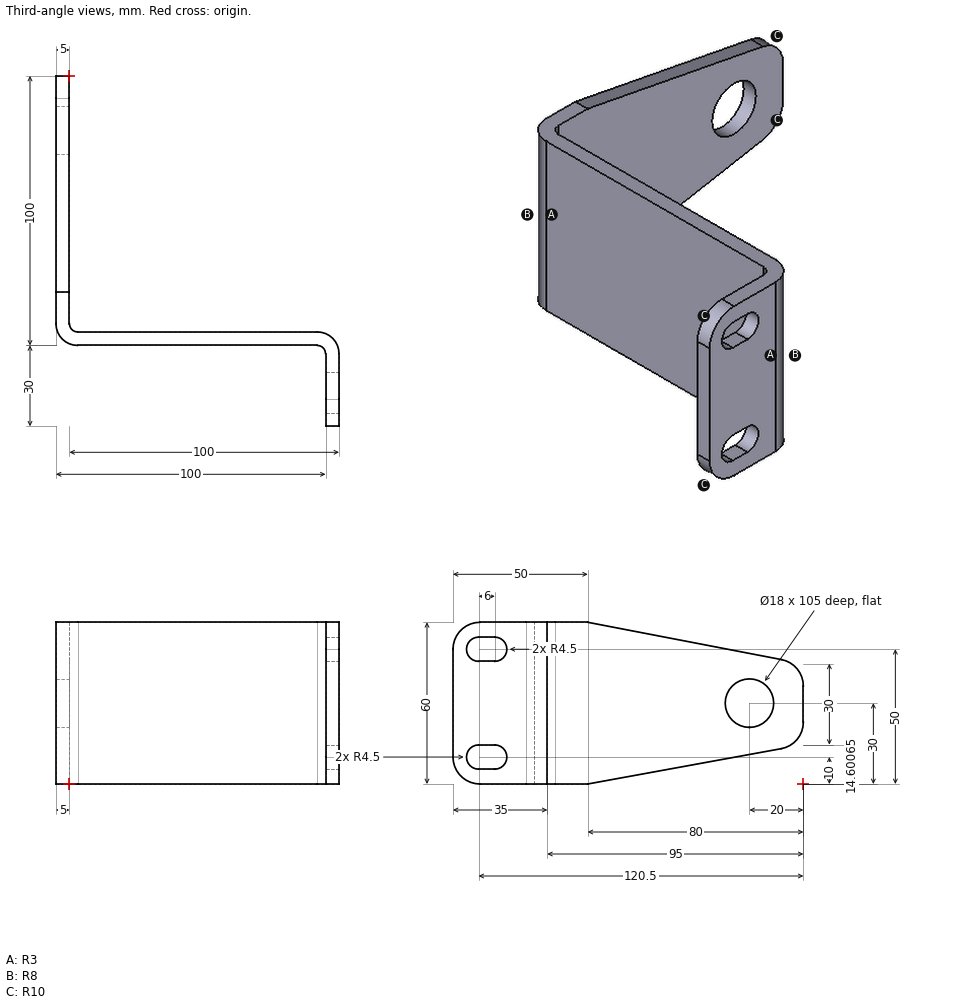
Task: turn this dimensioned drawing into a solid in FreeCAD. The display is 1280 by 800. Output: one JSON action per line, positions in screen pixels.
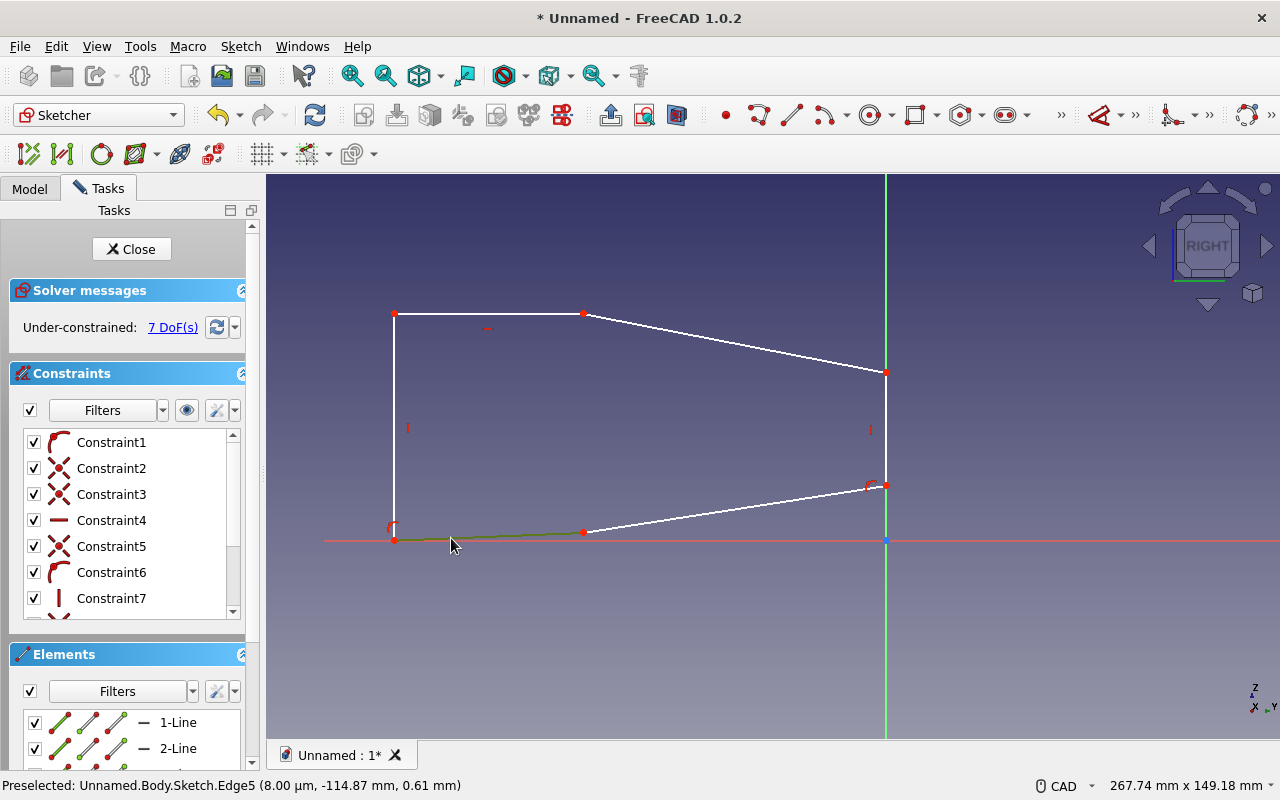
{"action": "key", "text": "h"}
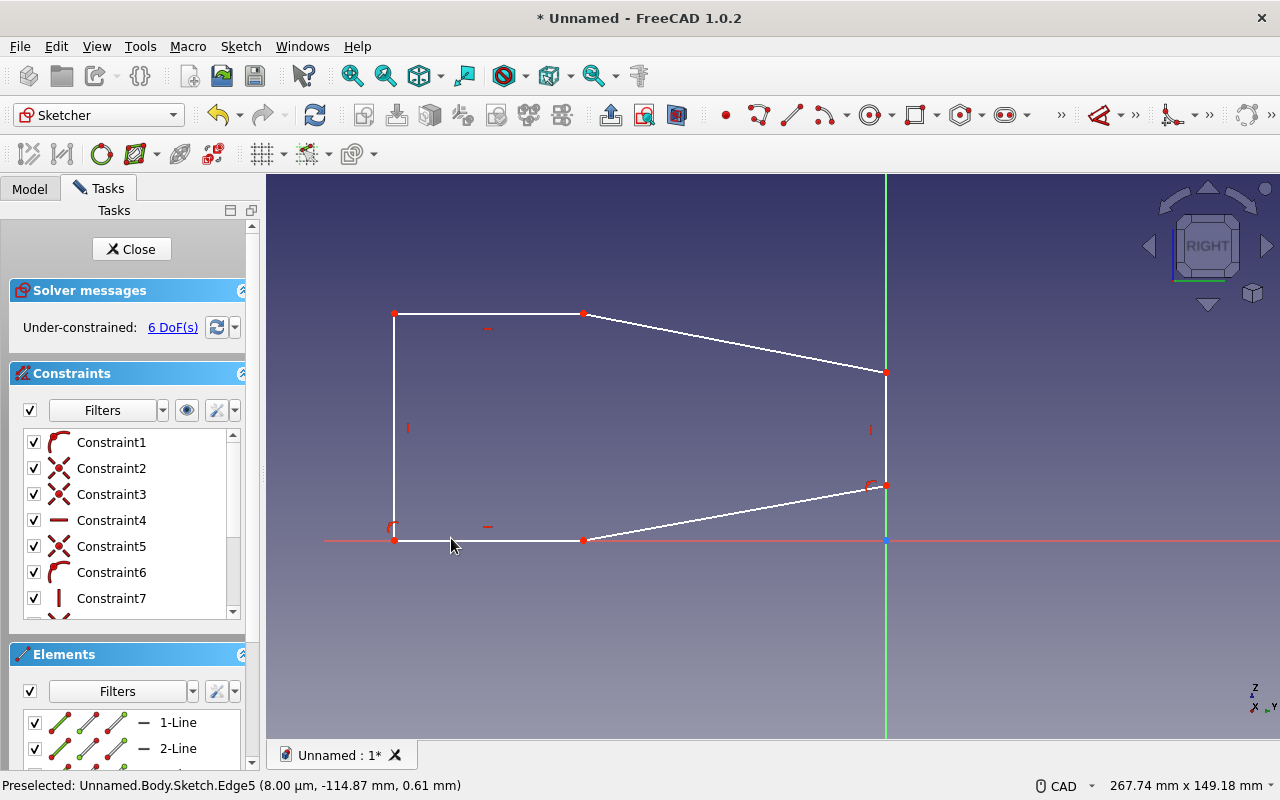
{"action": "left_click", "coordinate": [886, 452]}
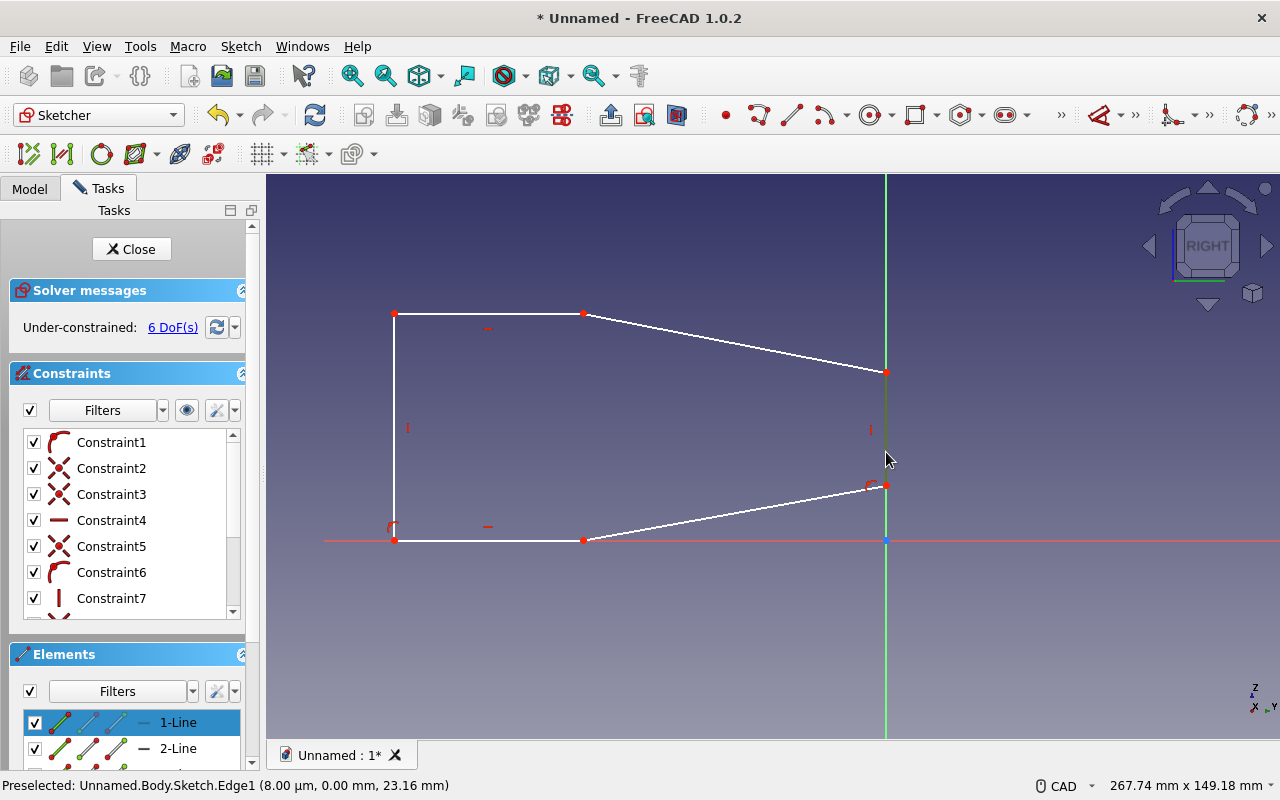
{"action": "left_click", "coordinate": [1120, 116]}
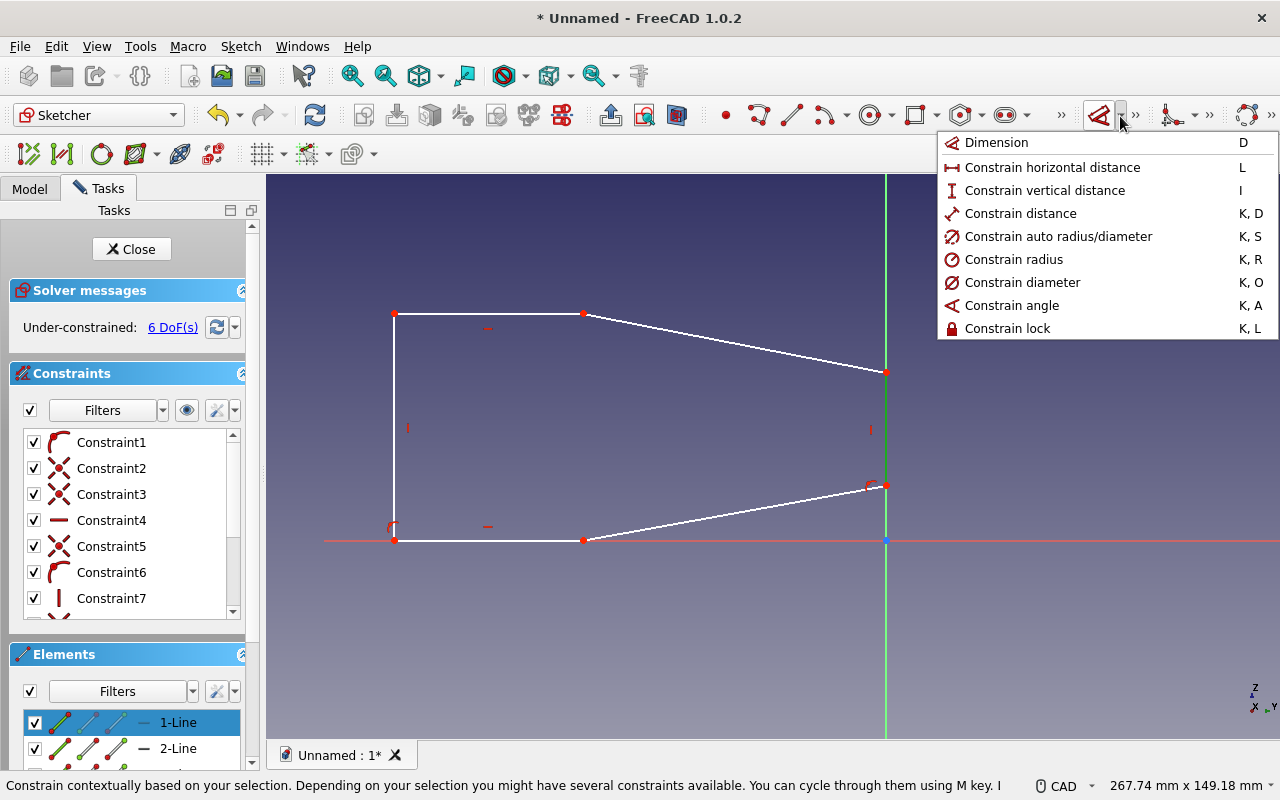
{"action": "left_click", "coordinate": [1108, 190]}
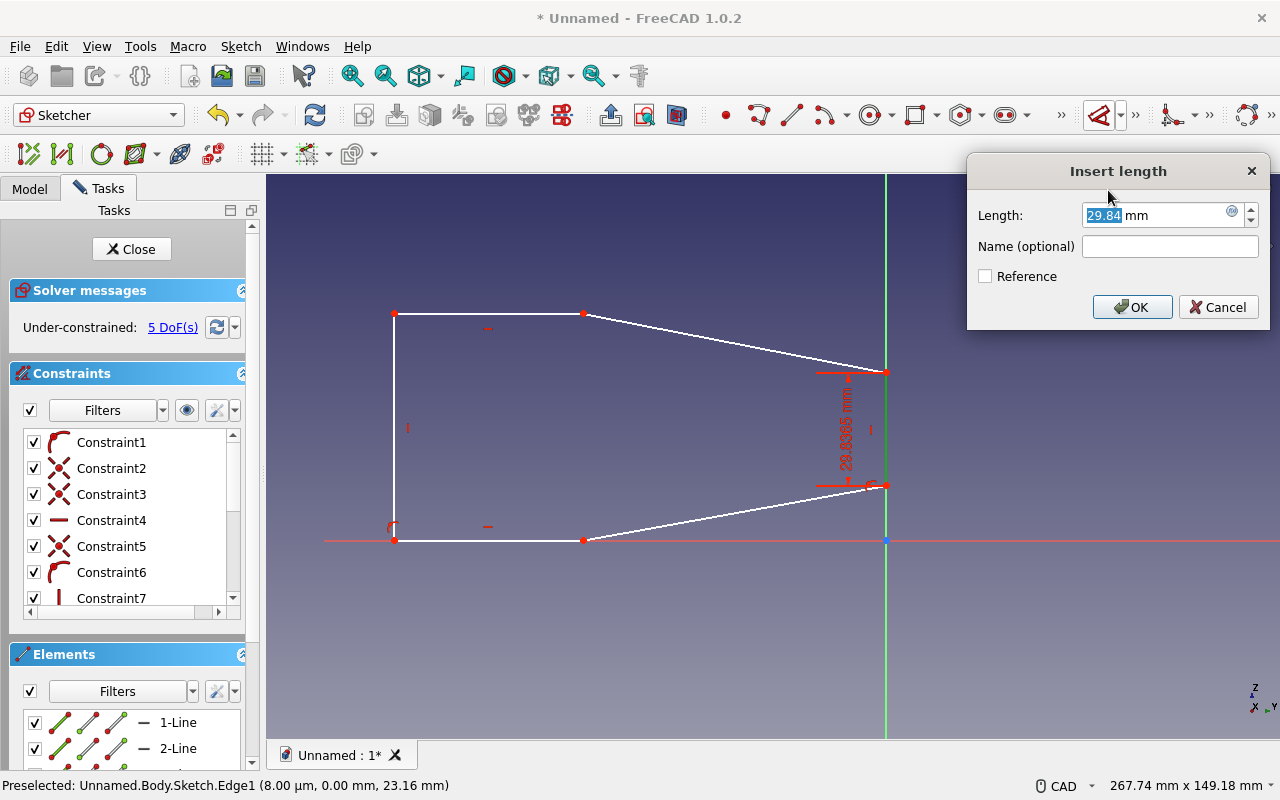
{"action": "type", "text": "30"}
{"action": "key", "text": "Return"}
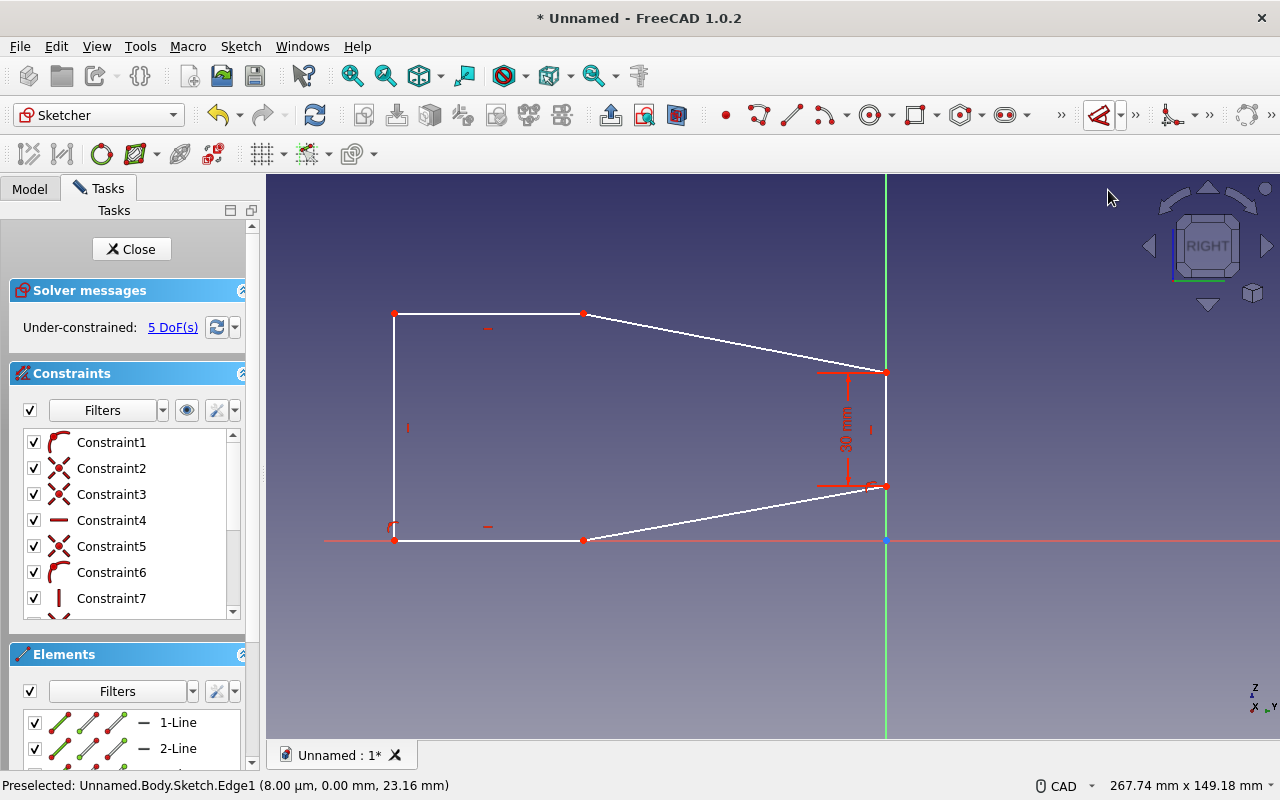
{"action": "left_click", "coordinate": [526, 314]}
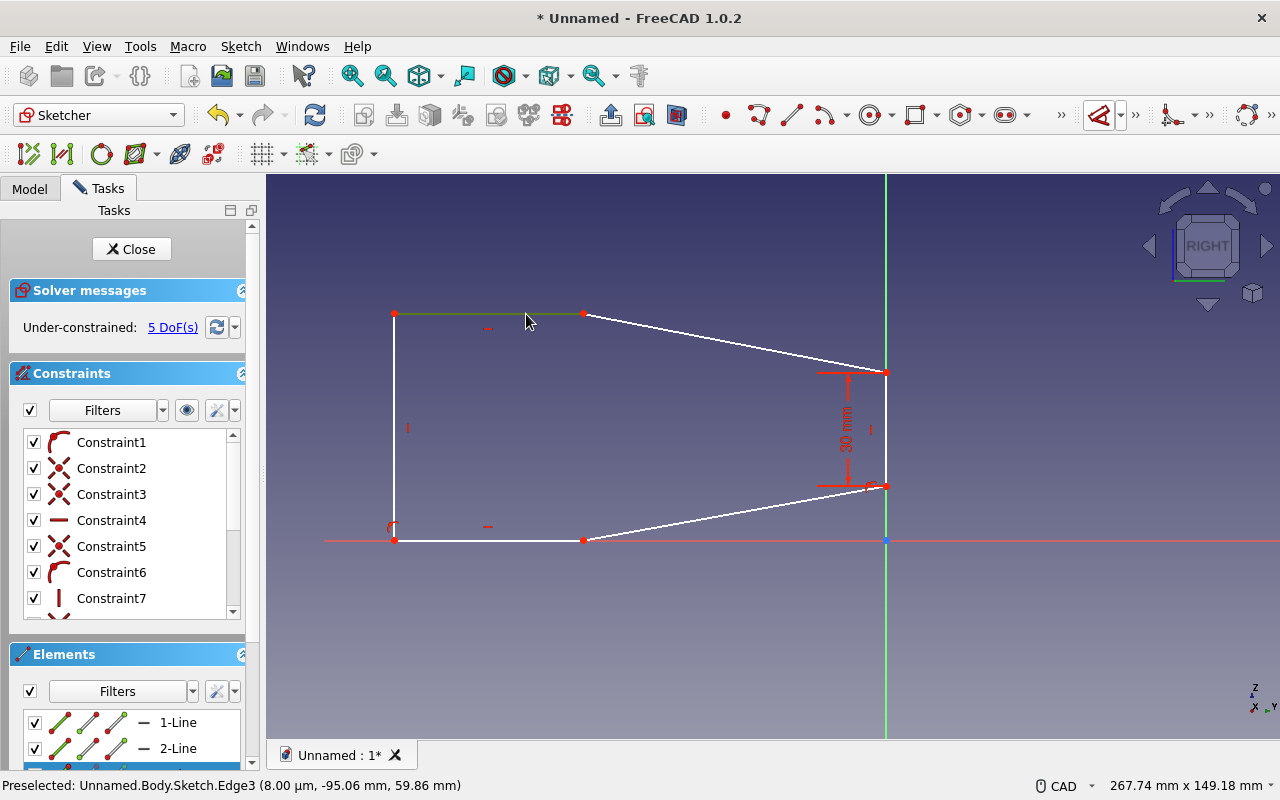
{"action": "key", "text": "l"}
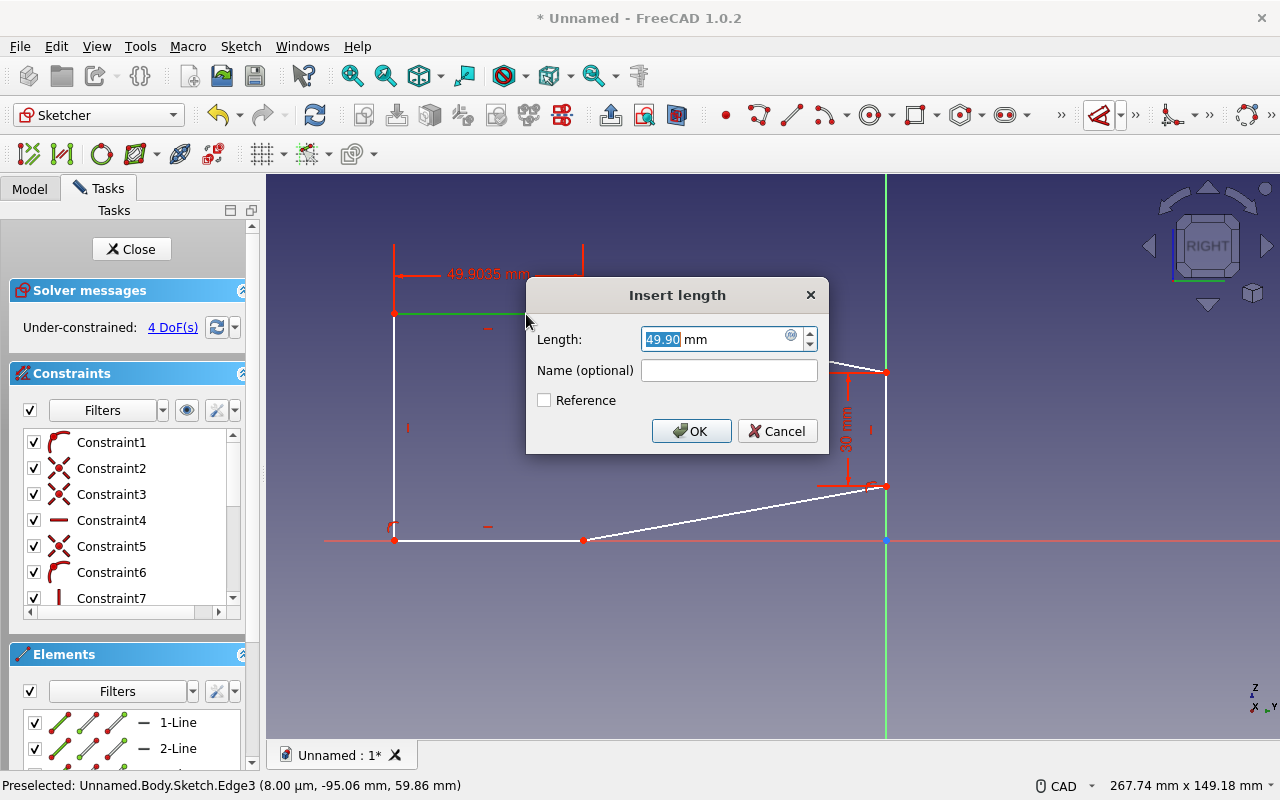
{"action": "type", "text": "50"}
{"action": "key", "text": "Return"}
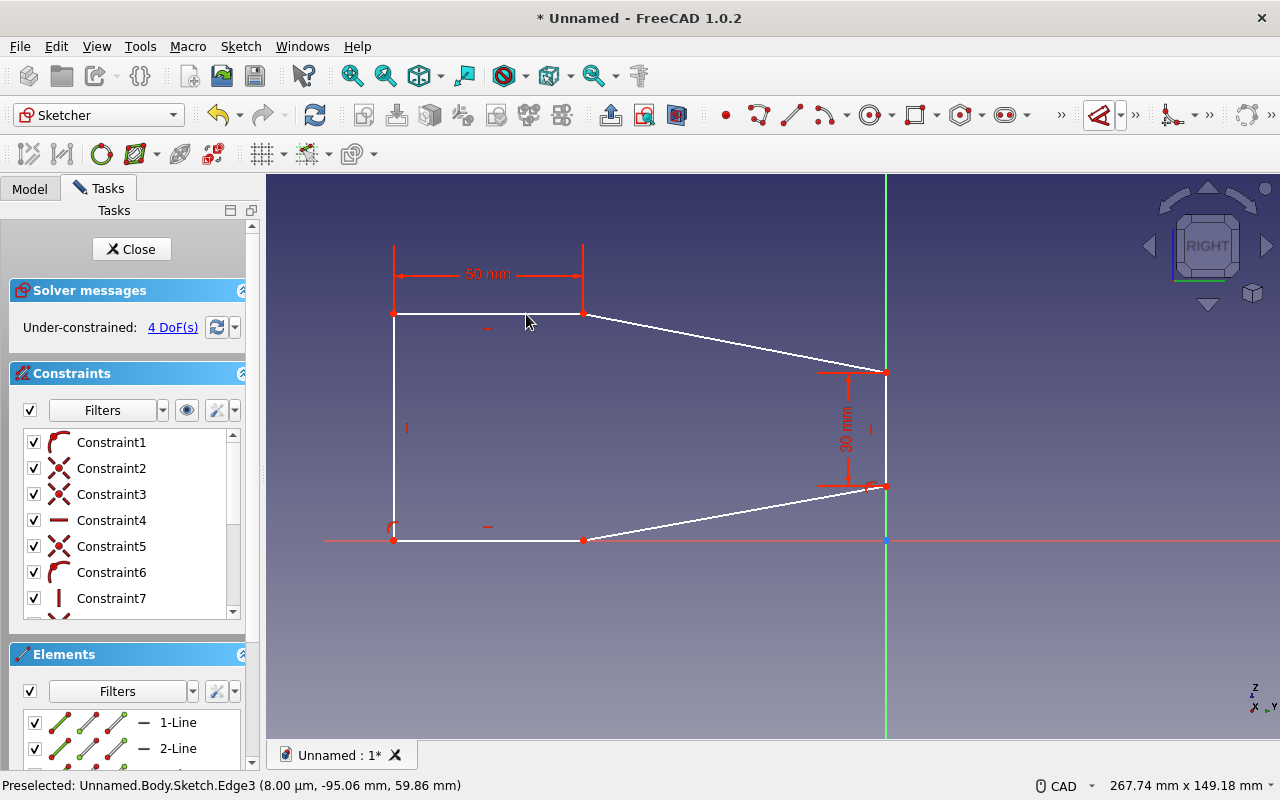
{"action": "left_click", "coordinate": [394, 382]}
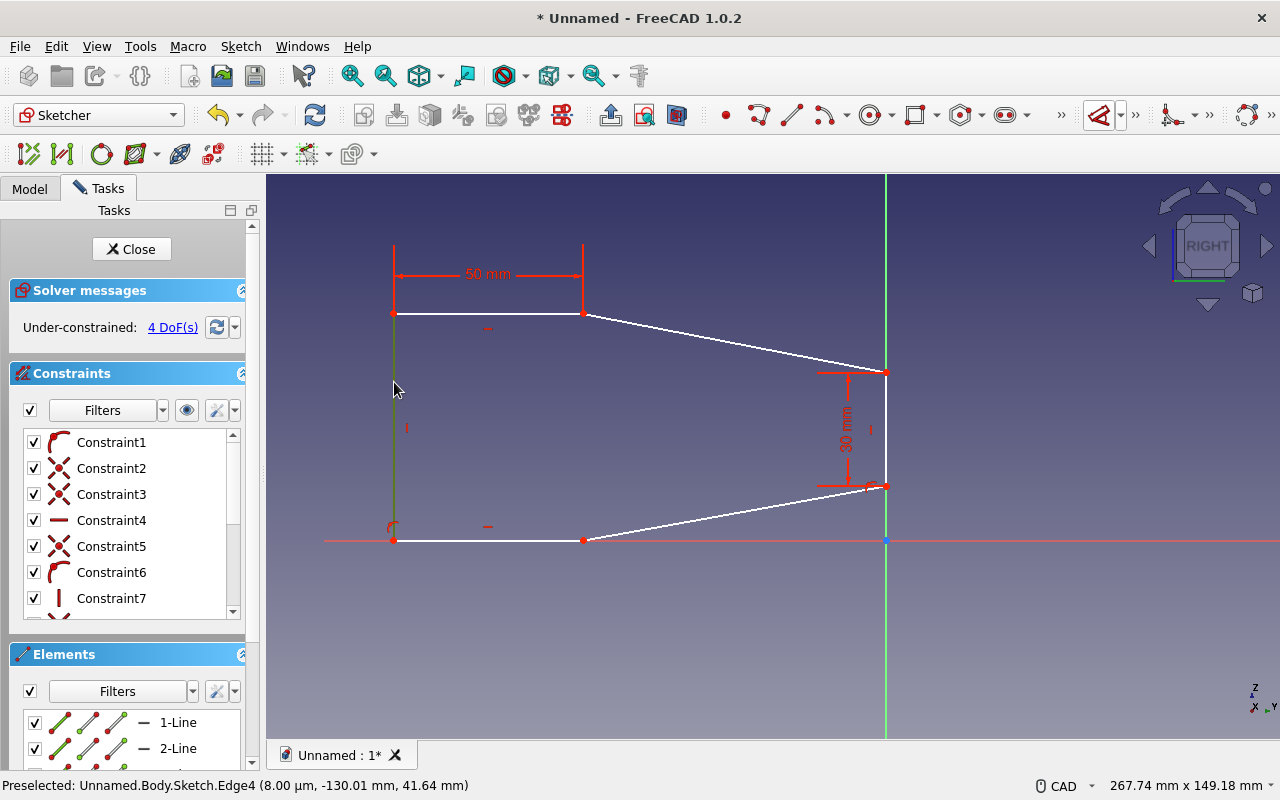
{"action": "key", "text": "i"}